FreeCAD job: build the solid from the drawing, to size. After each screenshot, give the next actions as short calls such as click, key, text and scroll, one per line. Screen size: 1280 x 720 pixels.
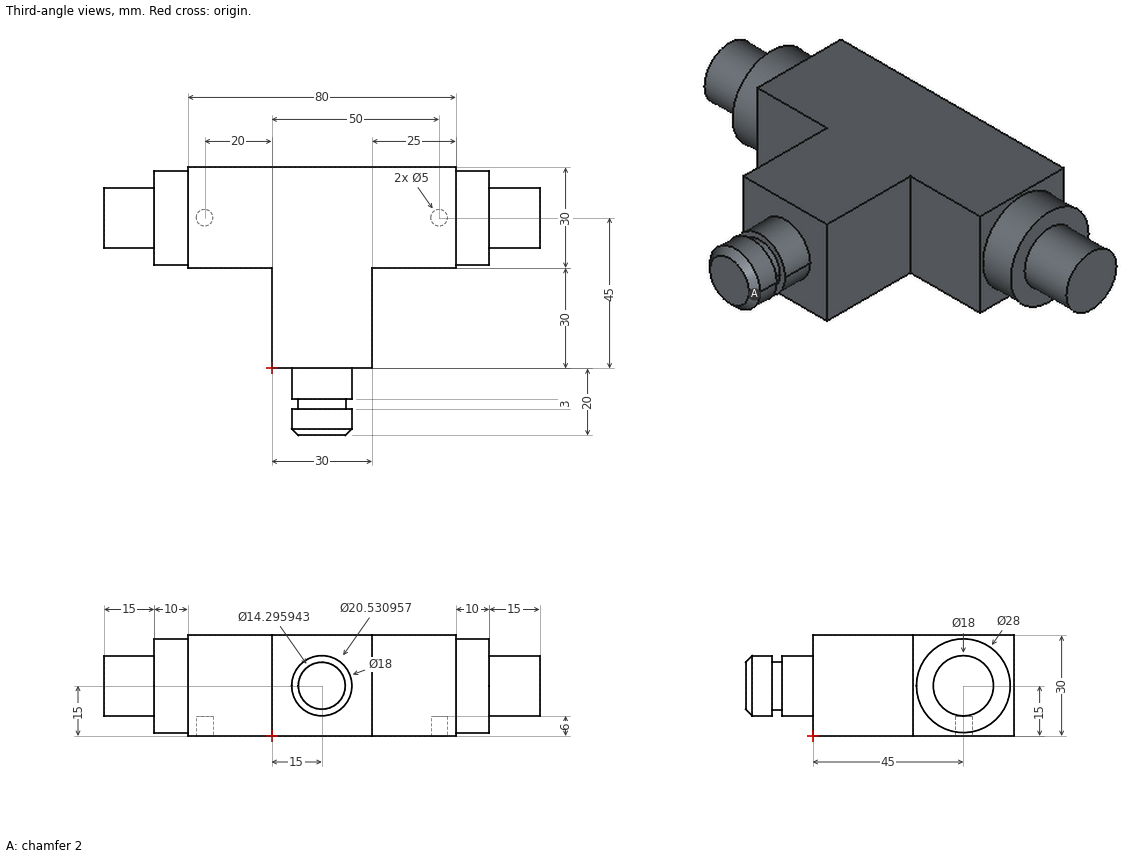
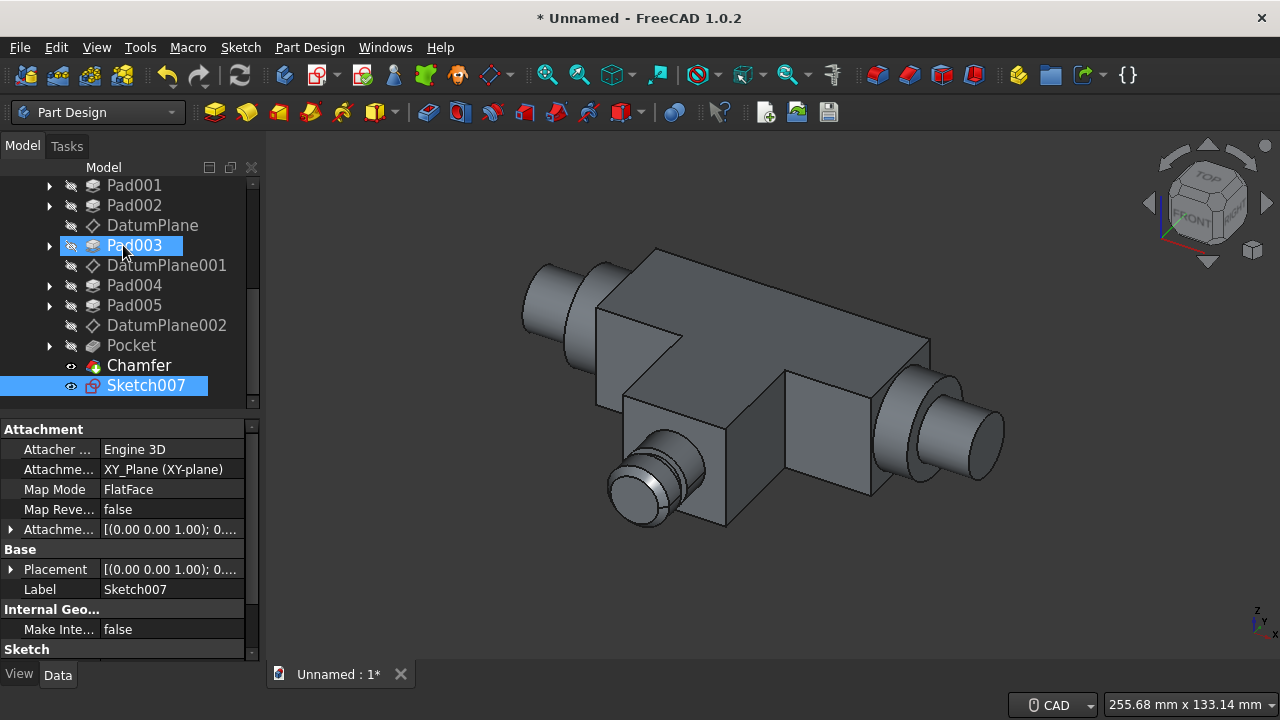
click(430, 112)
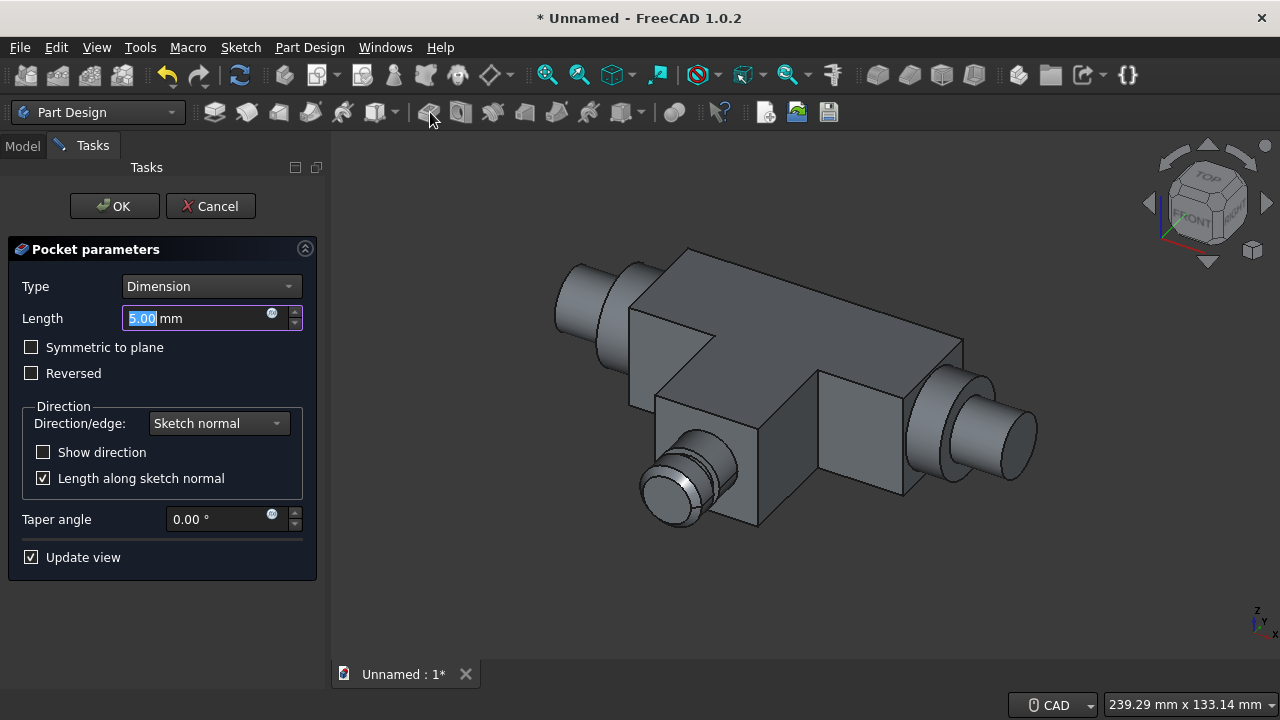
text(6)
key(Tab)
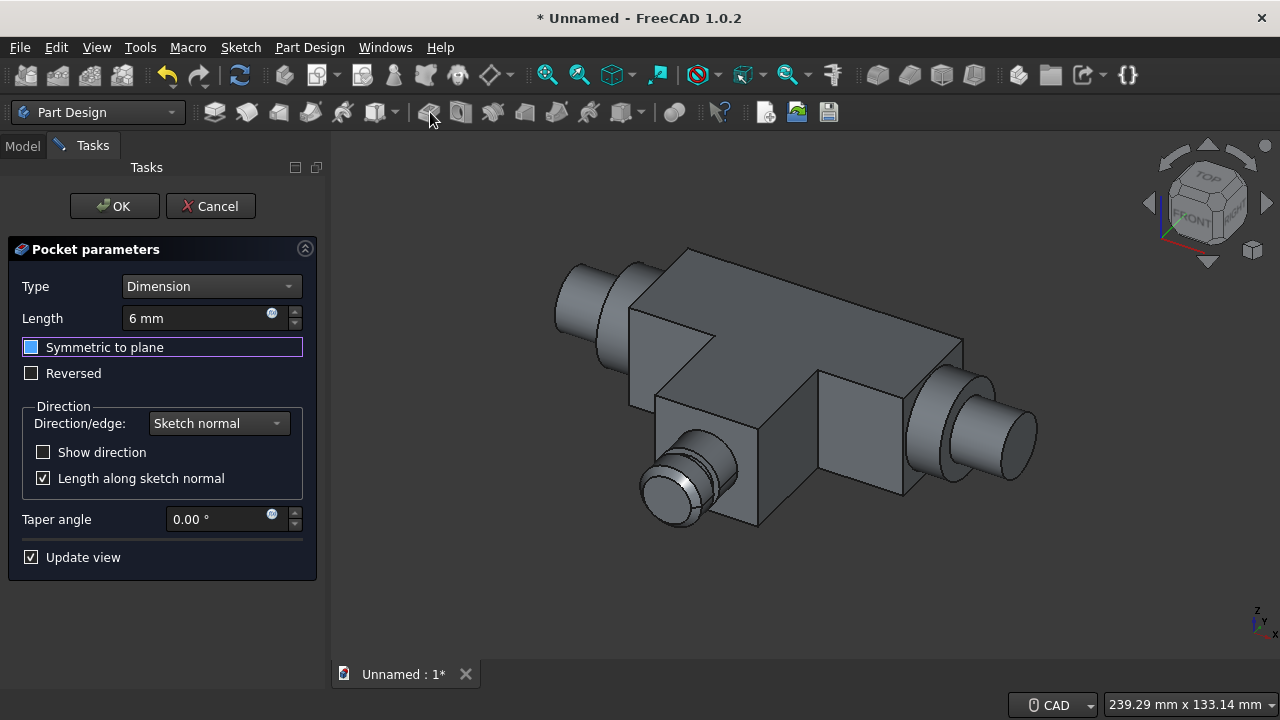
click(30, 373)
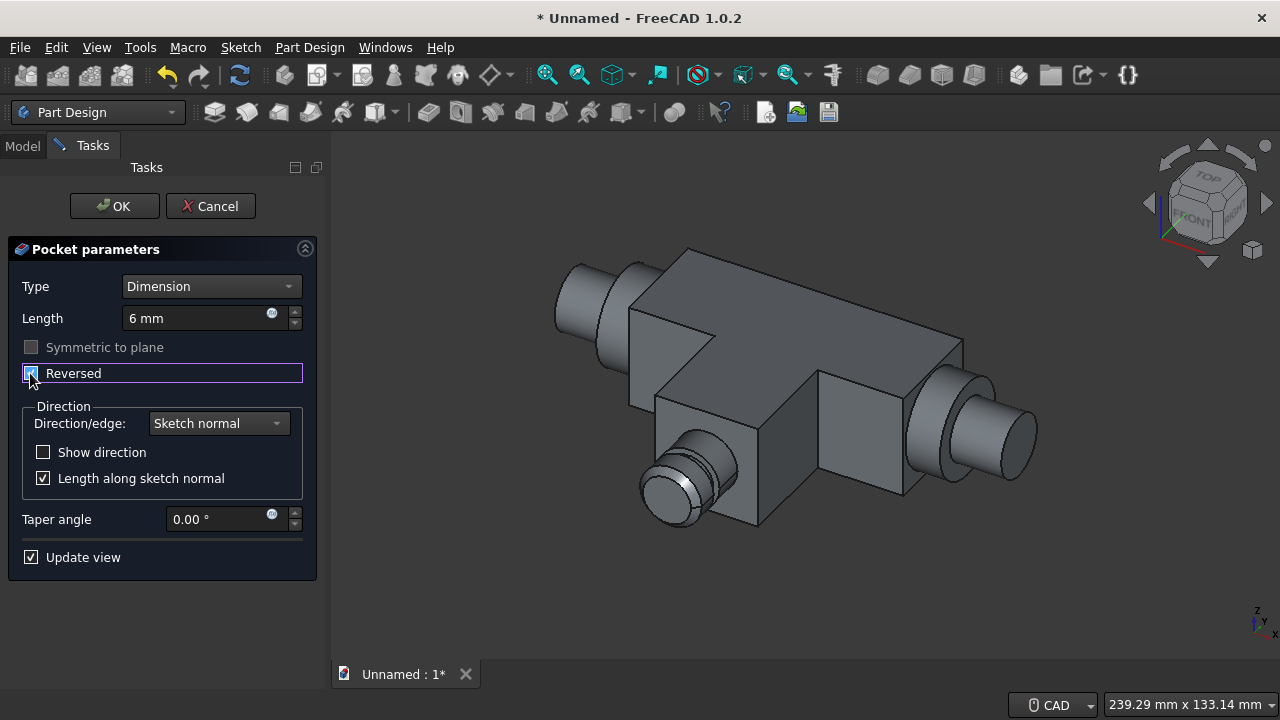
click(115, 206)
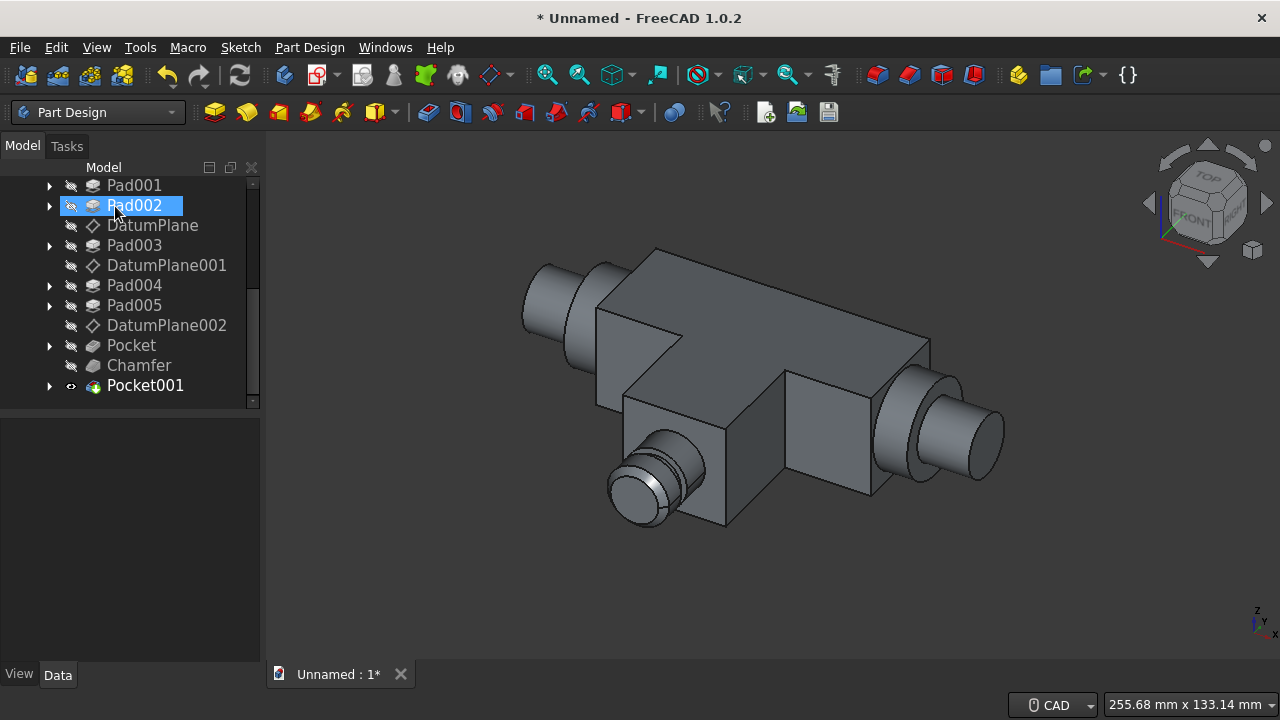
key(0)